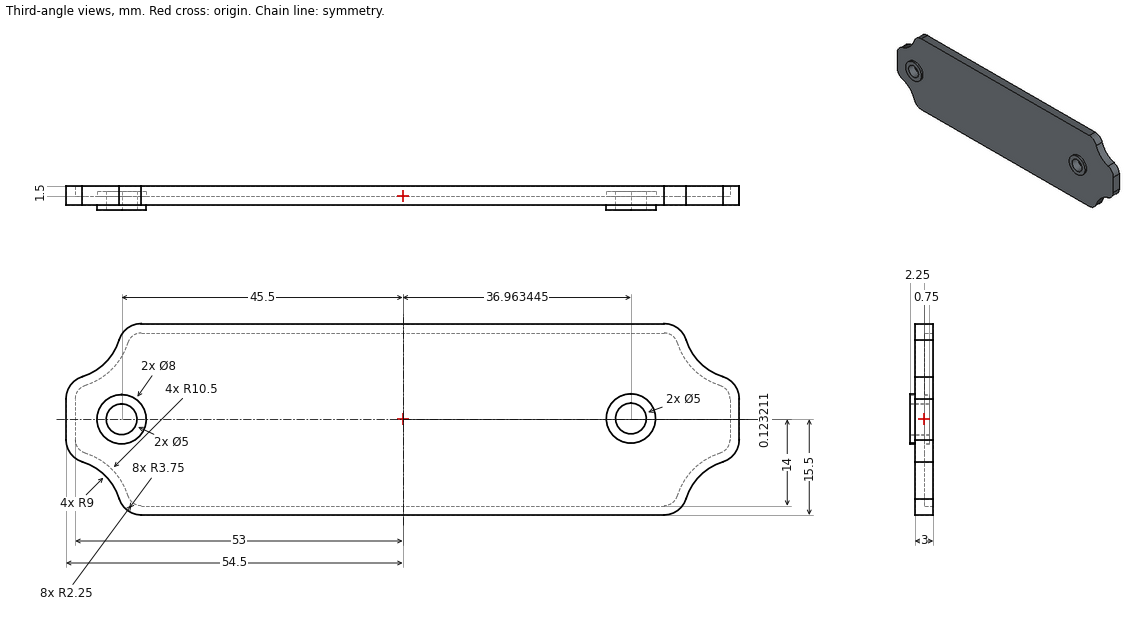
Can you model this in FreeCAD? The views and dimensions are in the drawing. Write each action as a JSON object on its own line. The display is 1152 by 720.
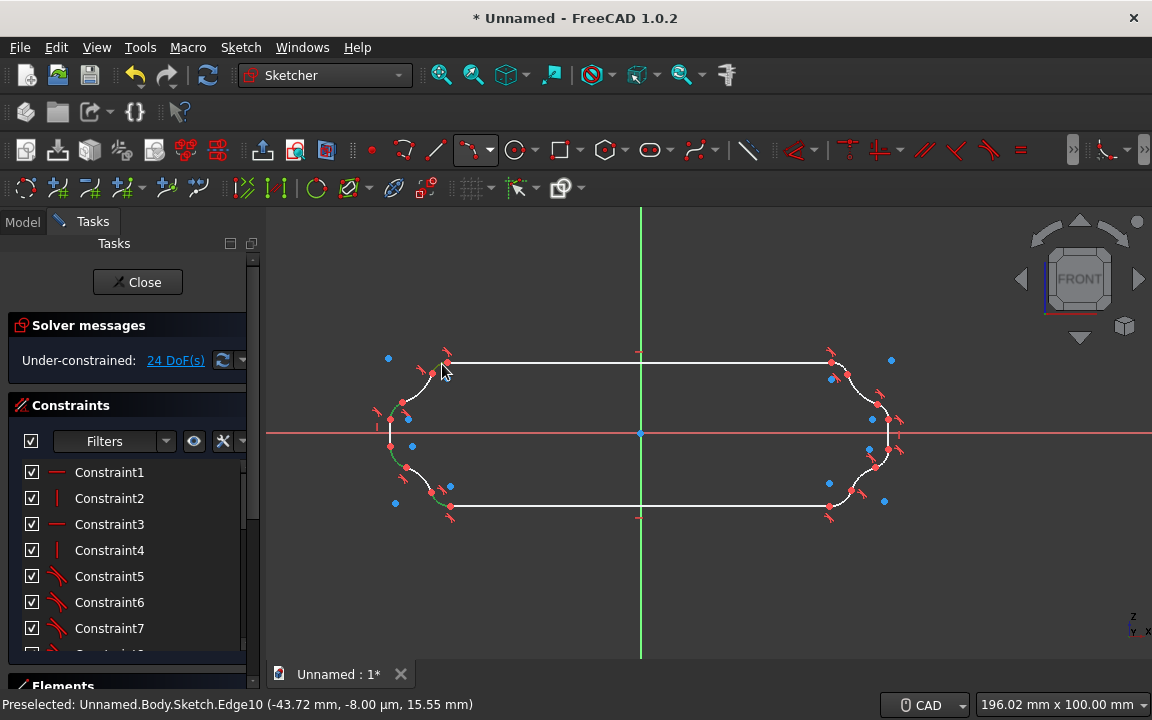
{"action": "scroll", "coordinate": [845, 369], "scroll_direction": "up", "scroll_amount": 4}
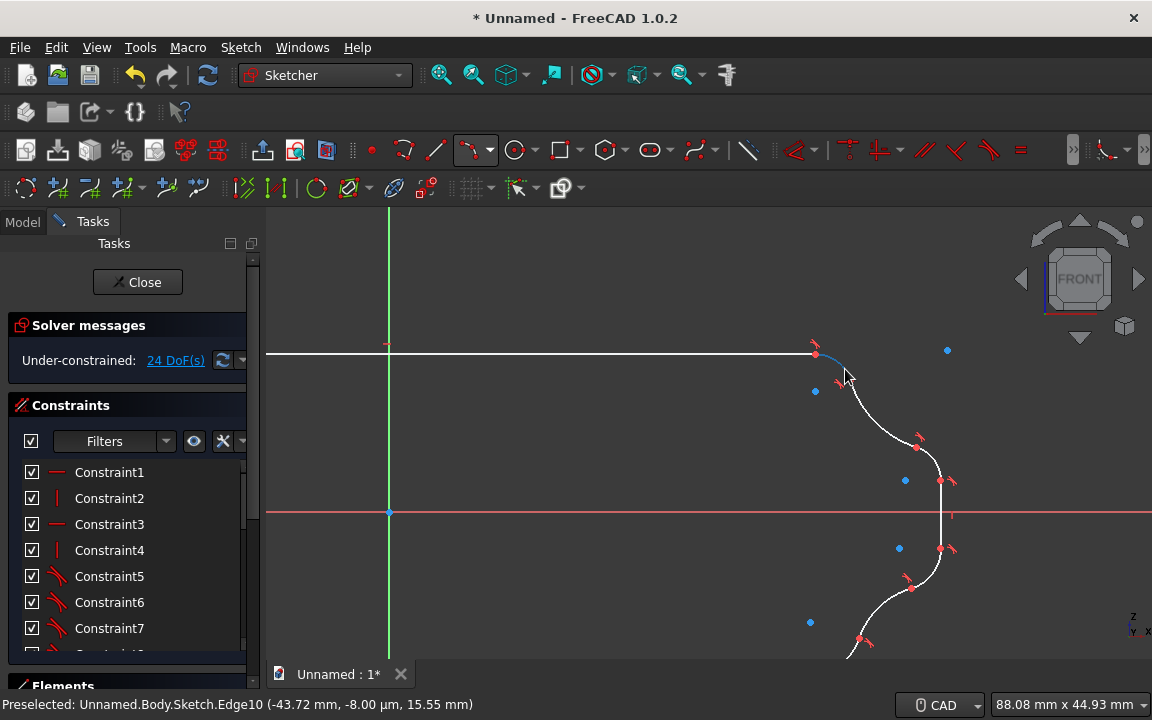
{"action": "left_click", "coordinate": [844, 368]}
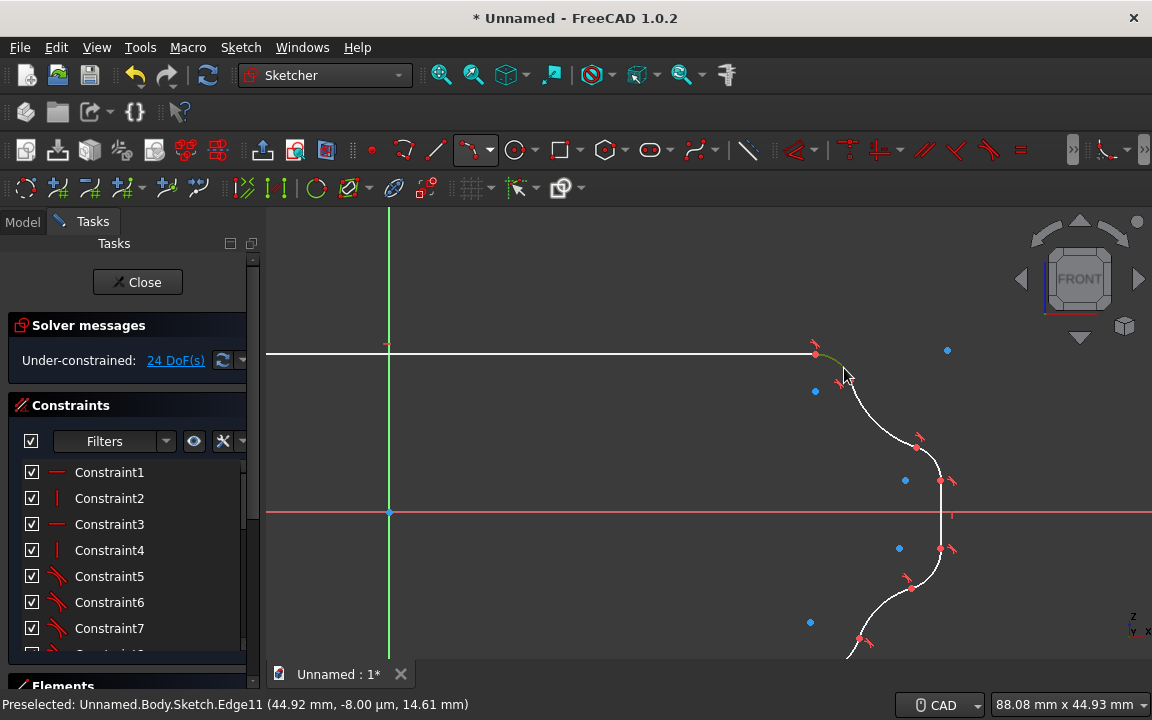
{"action": "left_click", "coordinate": [938, 468]}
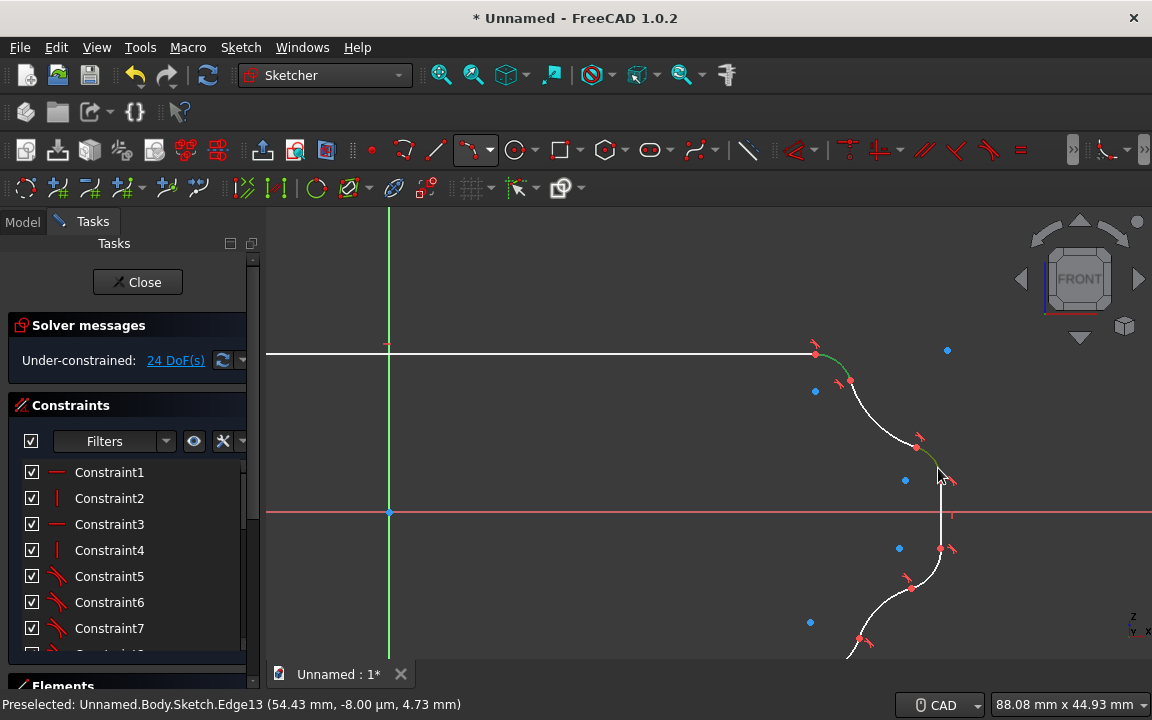
{"action": "left_click", "coordinate": [925, 581]}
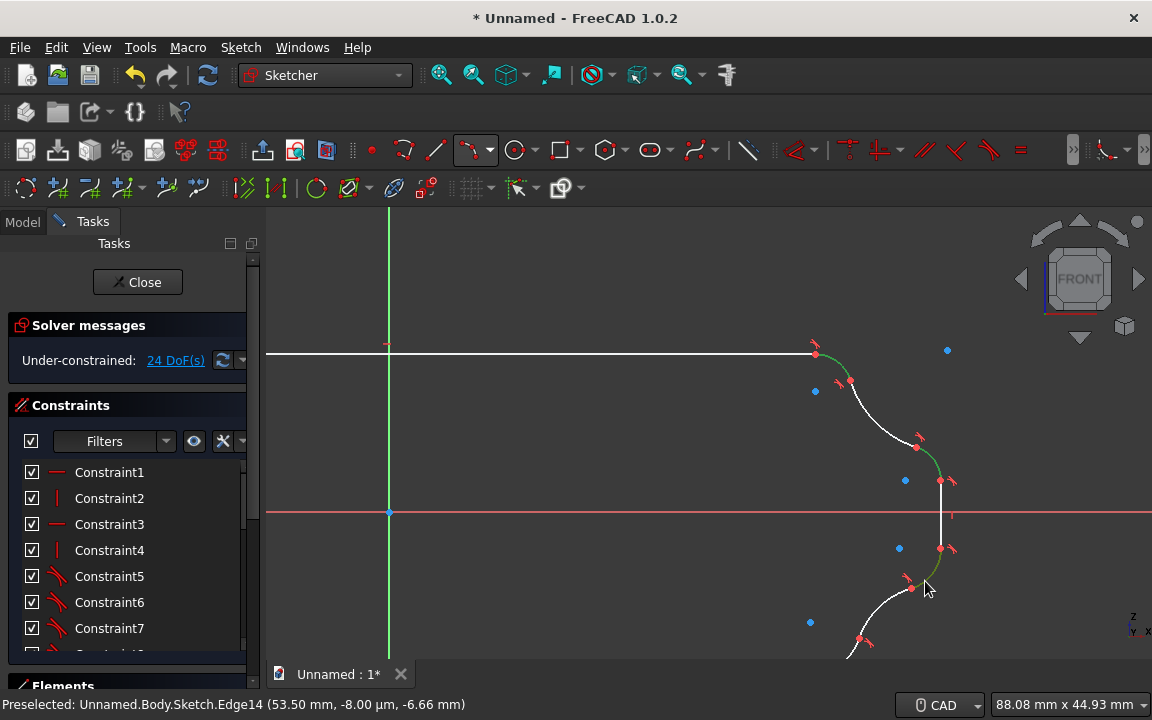
{"action": "scroll", "coordinate": [845, 368], "scroll_direction": "down", "scroll_amount": 4}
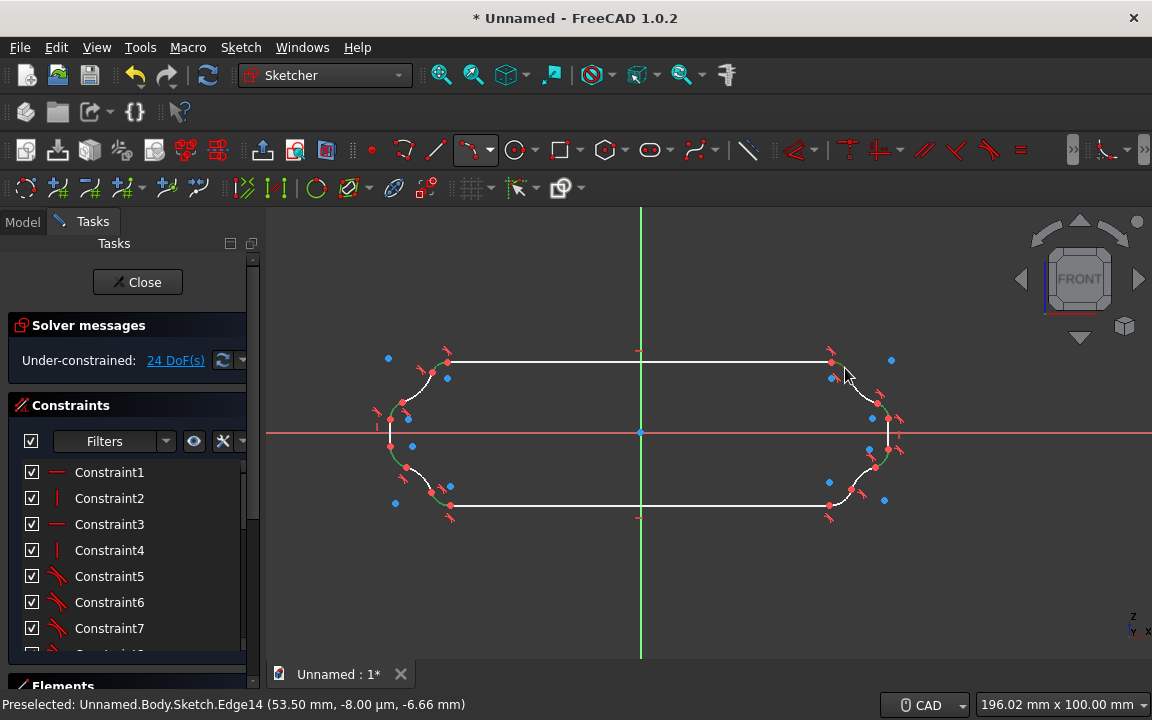
{"action": "scroll", "coordinate": [838, 504], "scroll_direction": "up", "scroll_amount": 3}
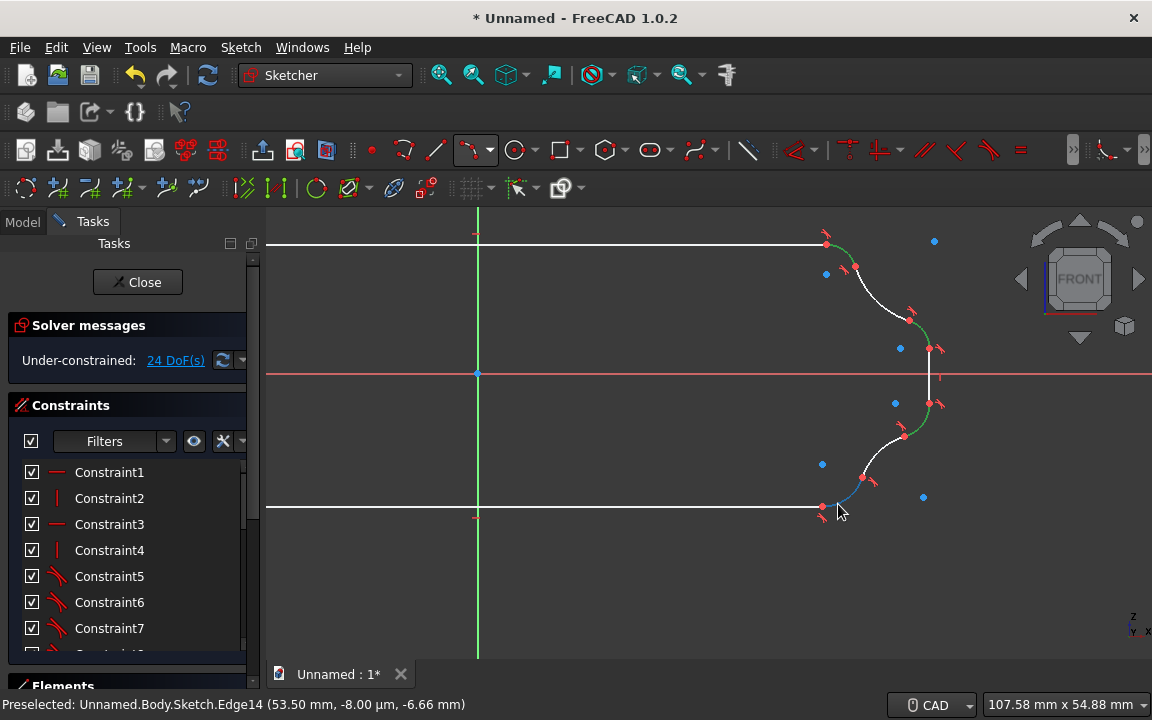
{"action": "left_click", "coordinate": [838, 504]}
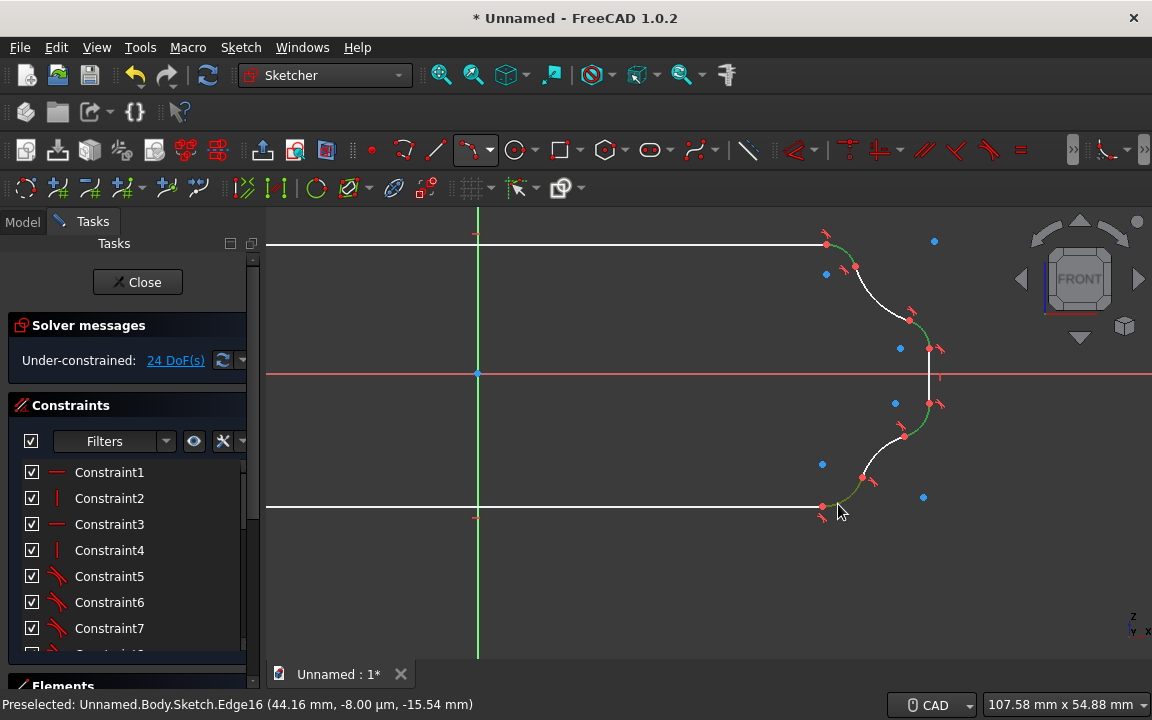
{"action": "left_click", "coordinate": [1022, 150]}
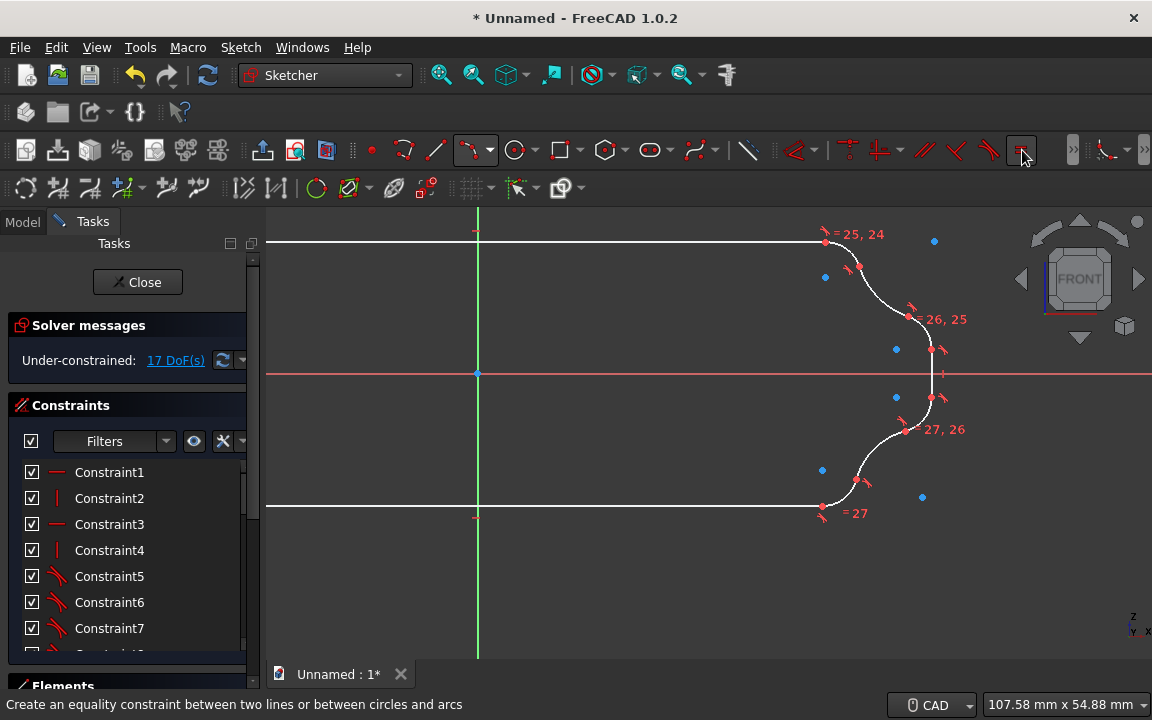
{"action": "scroll", "coordinate": [838, 505], "scroll_direction": "down", "scroll_amount": 3}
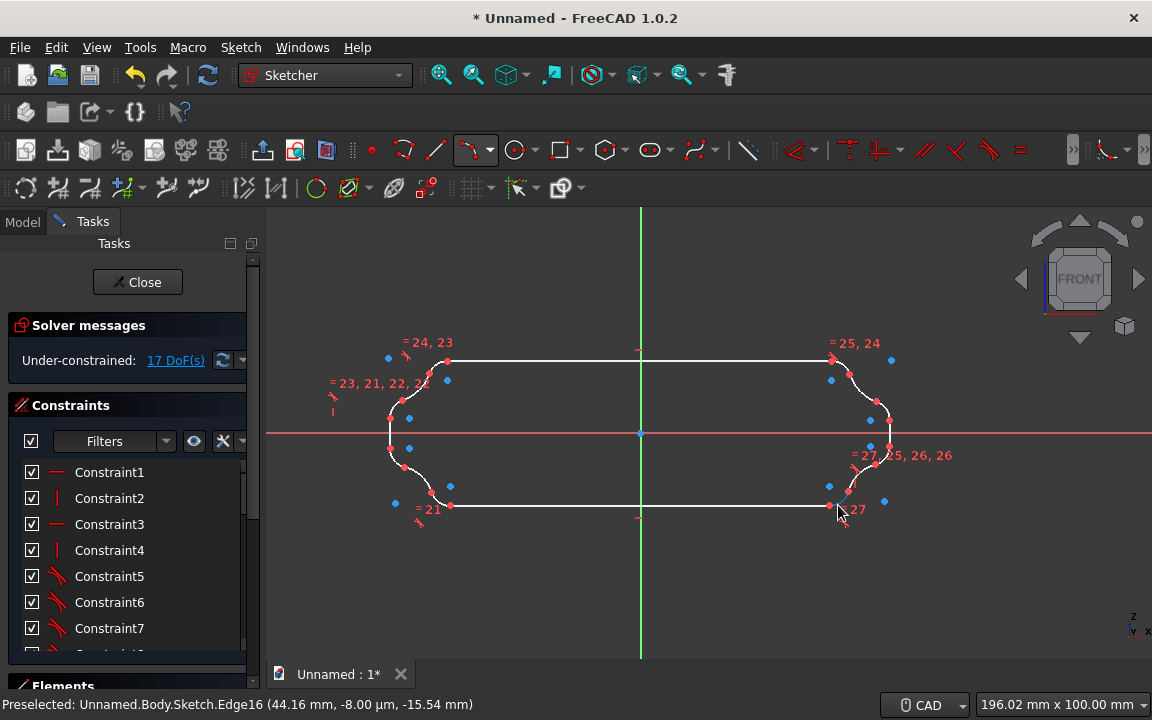
{"action": "left_click", "coordinate": [427, 482]}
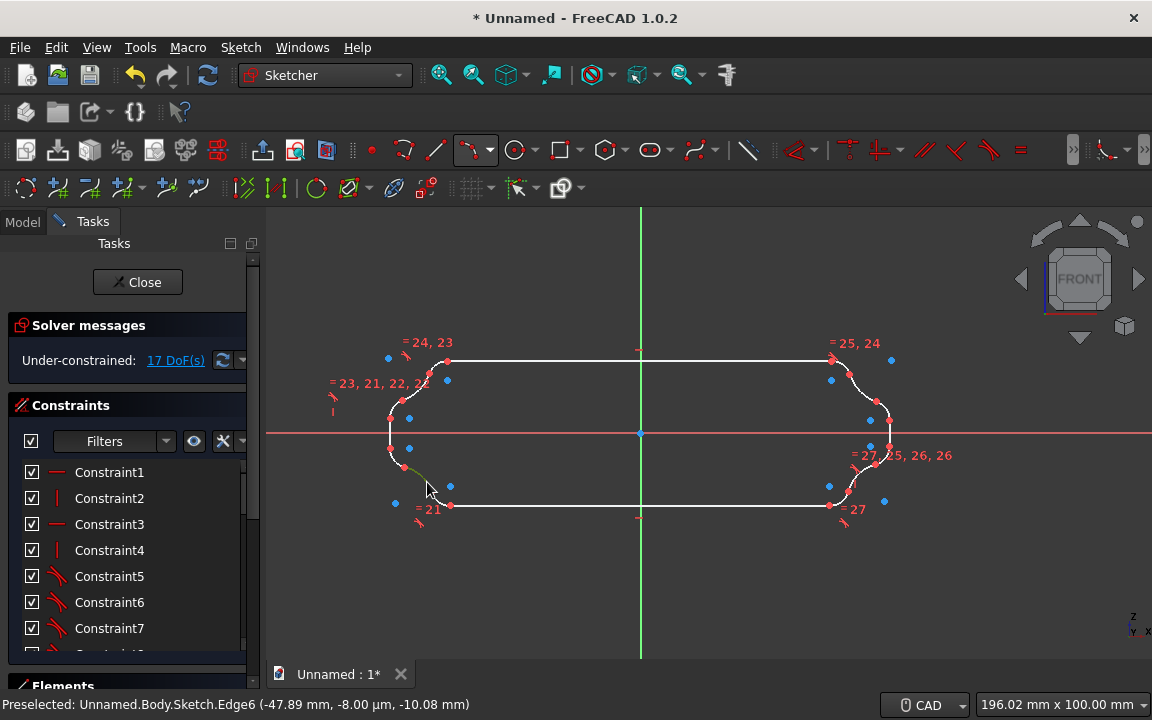
{"action": "scroll", "coordinate": [413, 395], "scroll_direction": "up", "scroll_amount": 4}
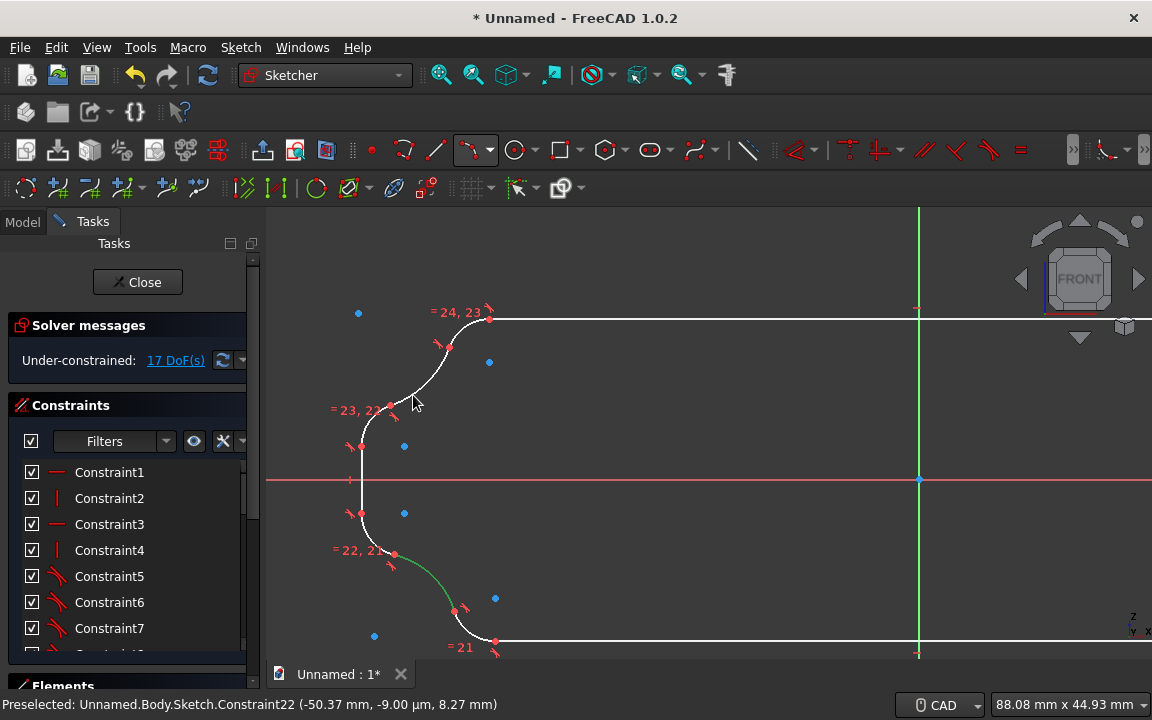
{"action": "left_click", "coordinate": [413, 394]}